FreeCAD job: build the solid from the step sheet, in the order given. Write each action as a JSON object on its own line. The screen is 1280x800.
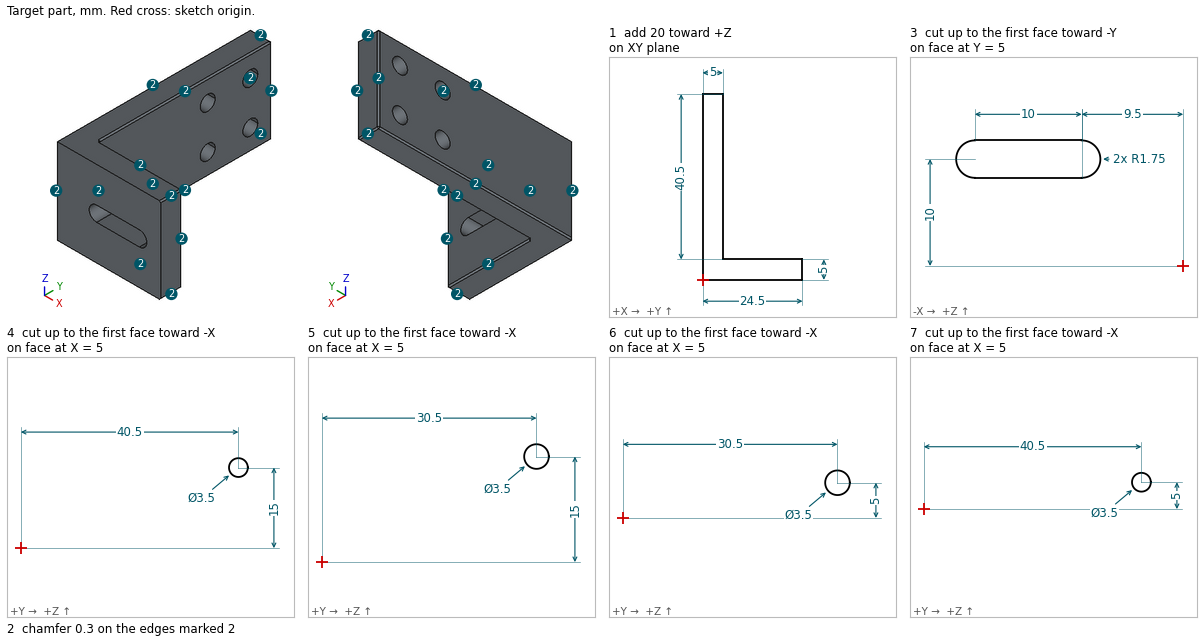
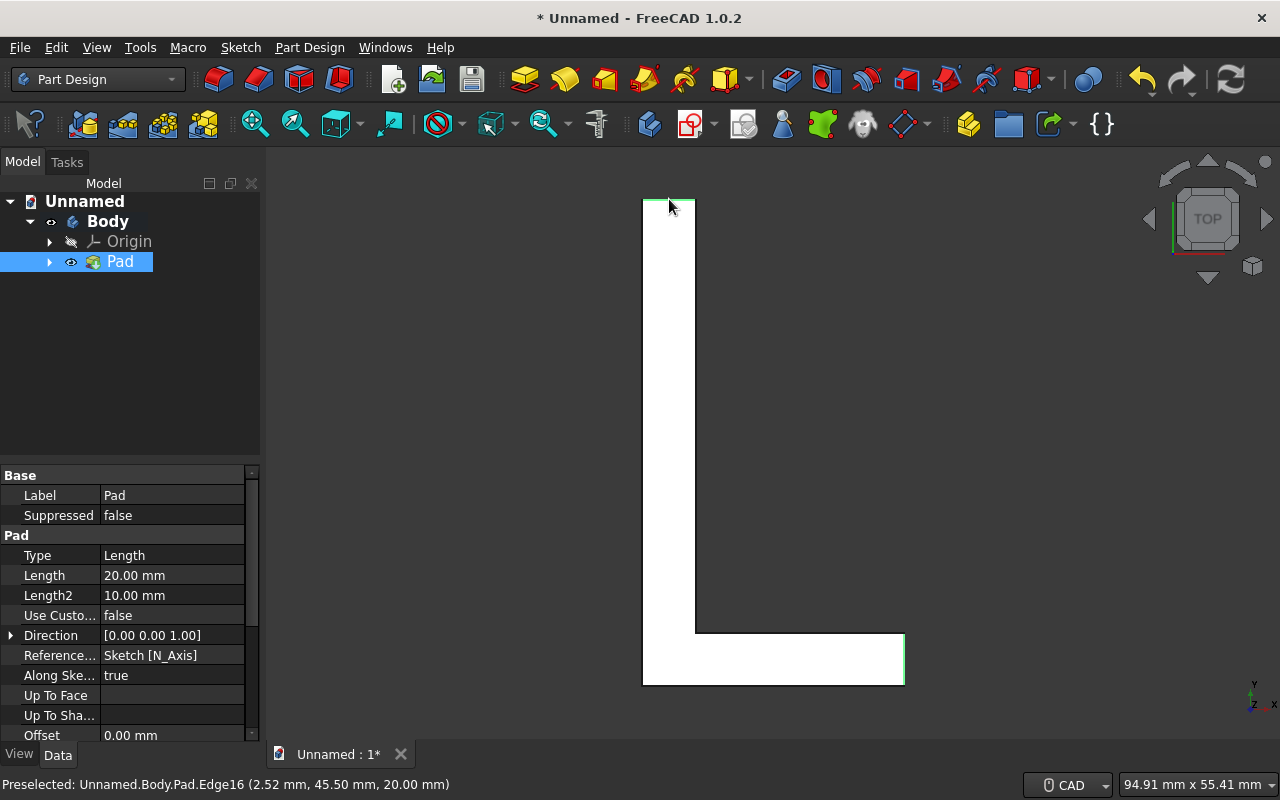
{"action": "key", "text": "1"}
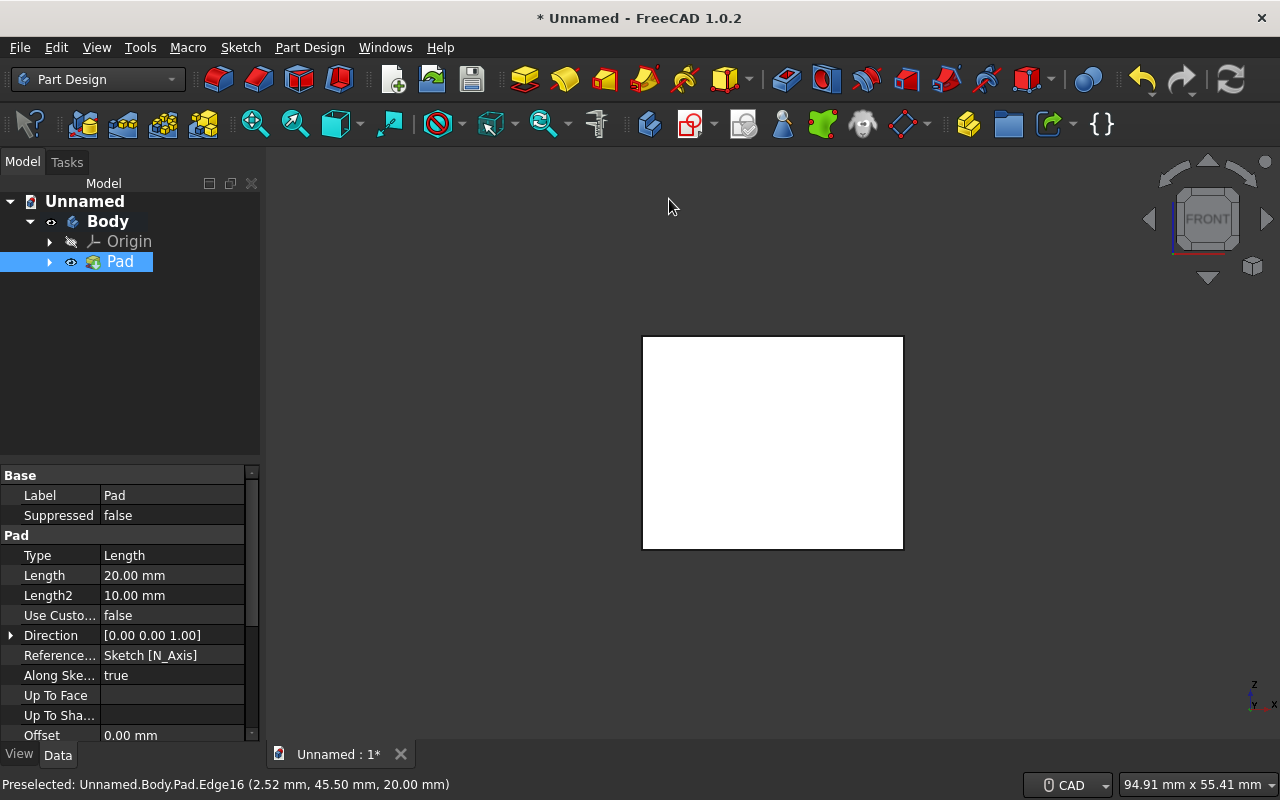
{"action": "left_click", "coordinate": [256, 124]}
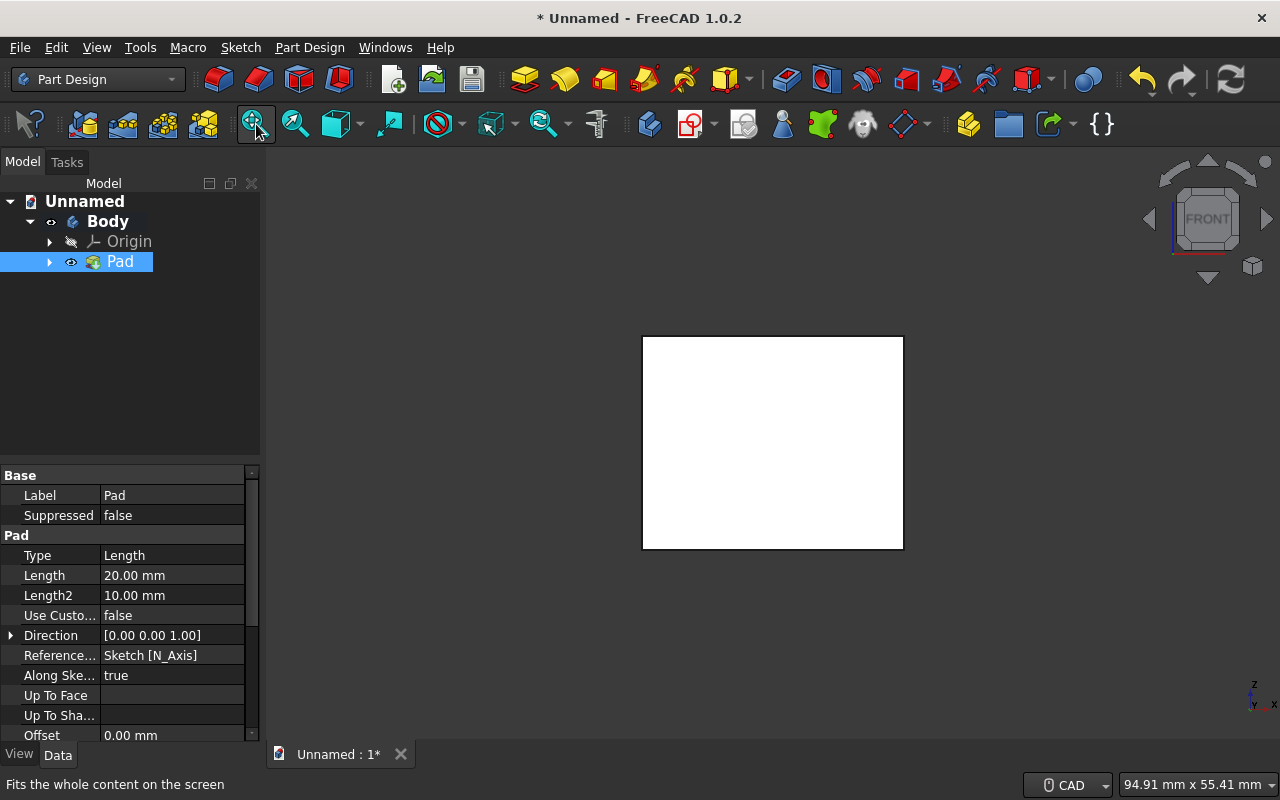
{"action": "key", "text": "3"}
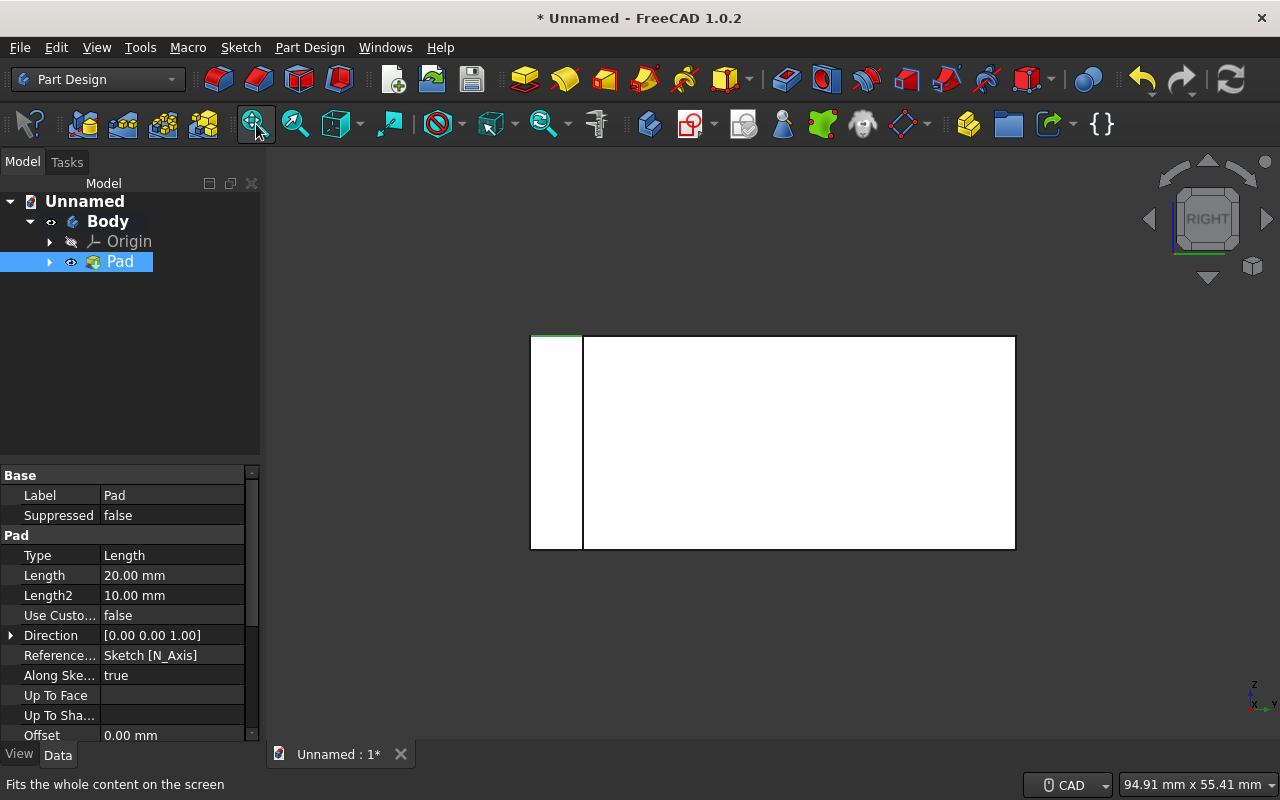
{"action": "left_click", "coordinate": [557, 549], "text": "ctrl"}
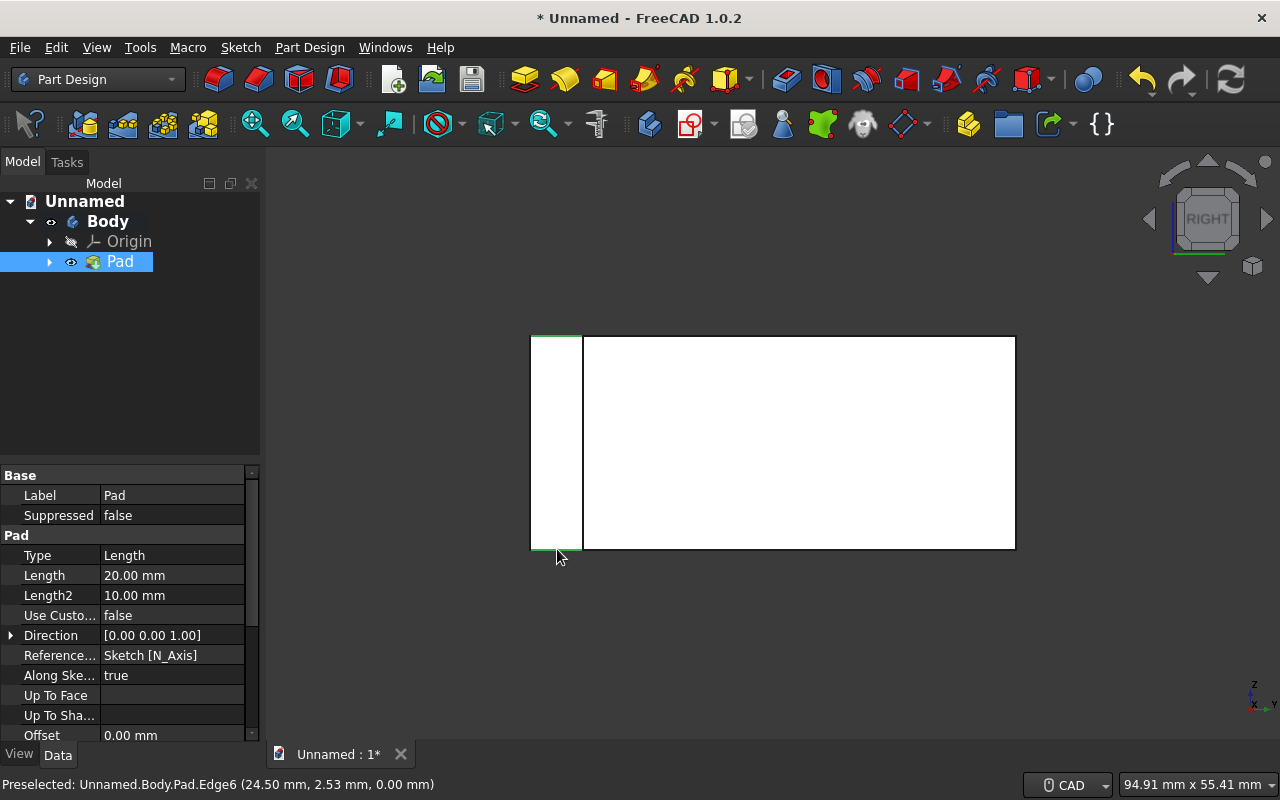
{"action": "key", "text": "5"}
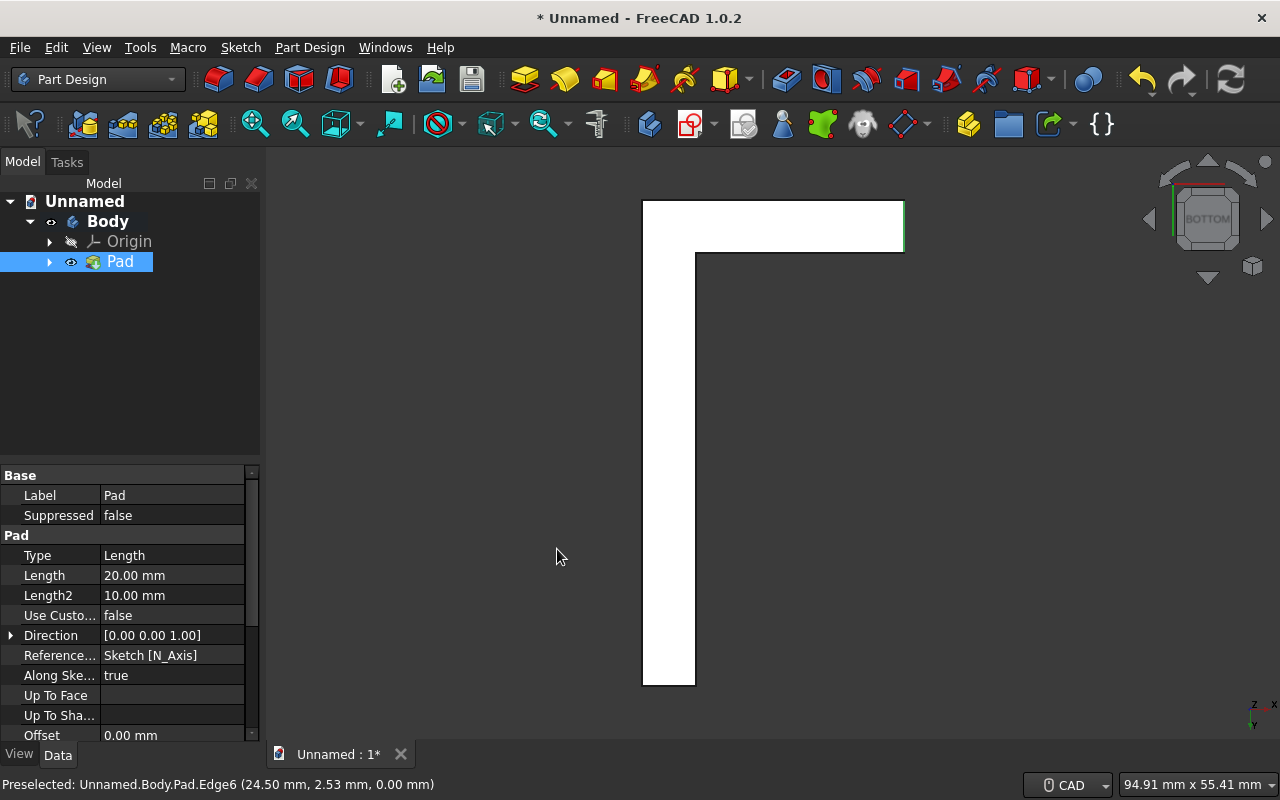
{"action": "left_click", "coordinate": [669, 685], "text": "ctrl"}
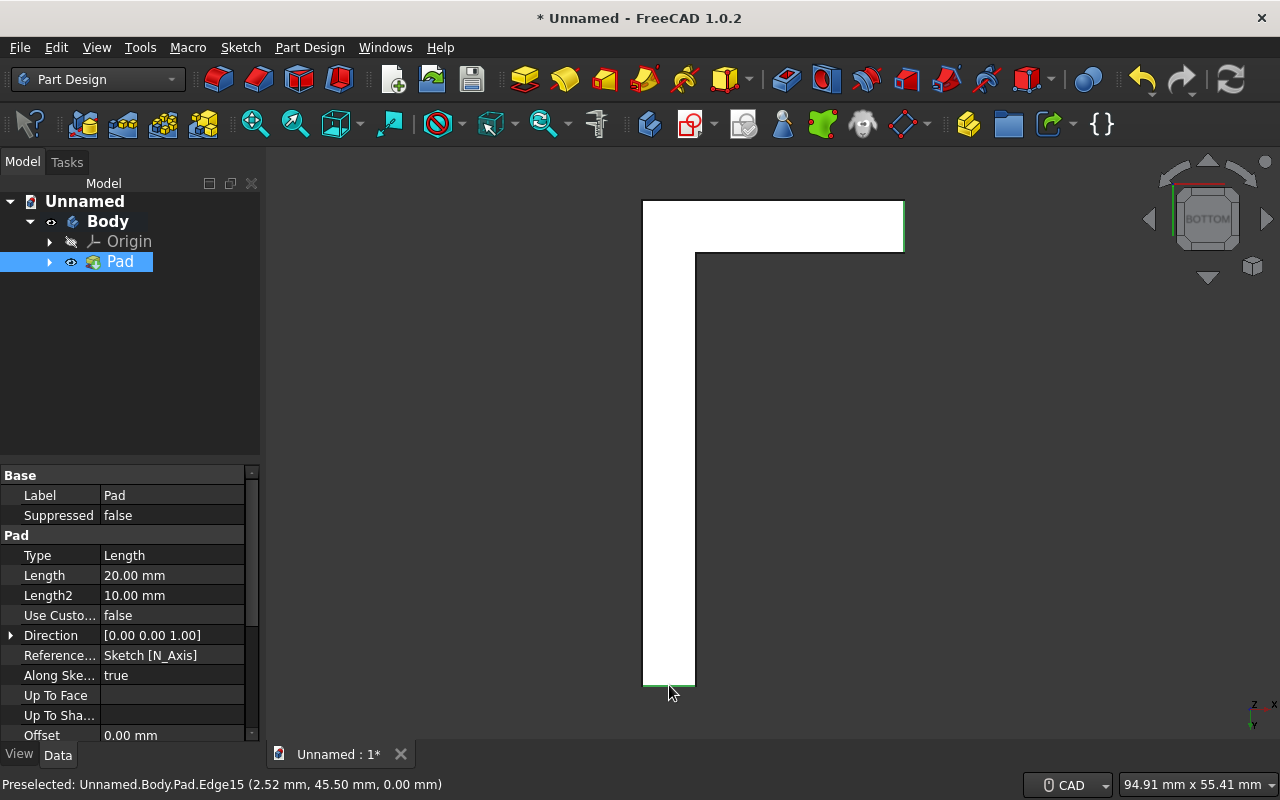
{"action": "key", "text": "4"}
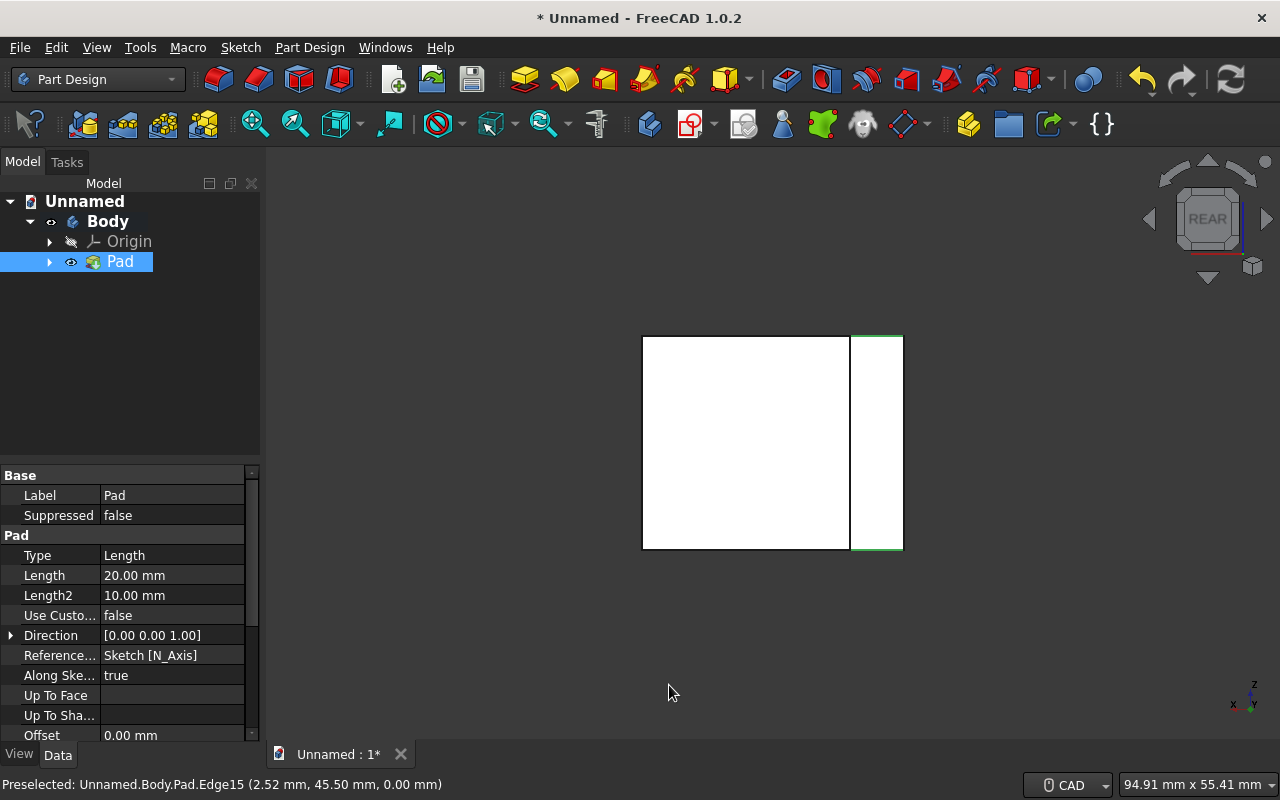
{"action": "key", "text": "v f"}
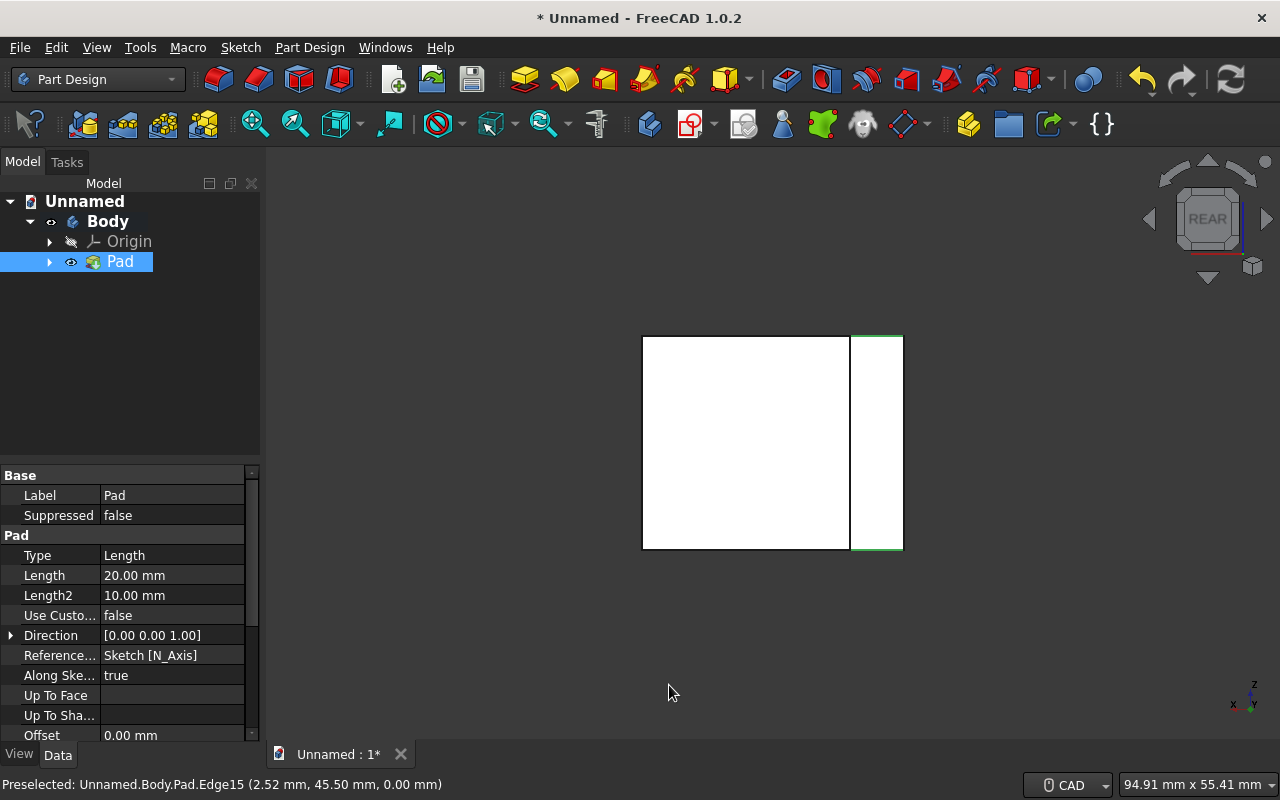
{"action": "left_click", "coordinate": [746, 442], "text": "ctrl"}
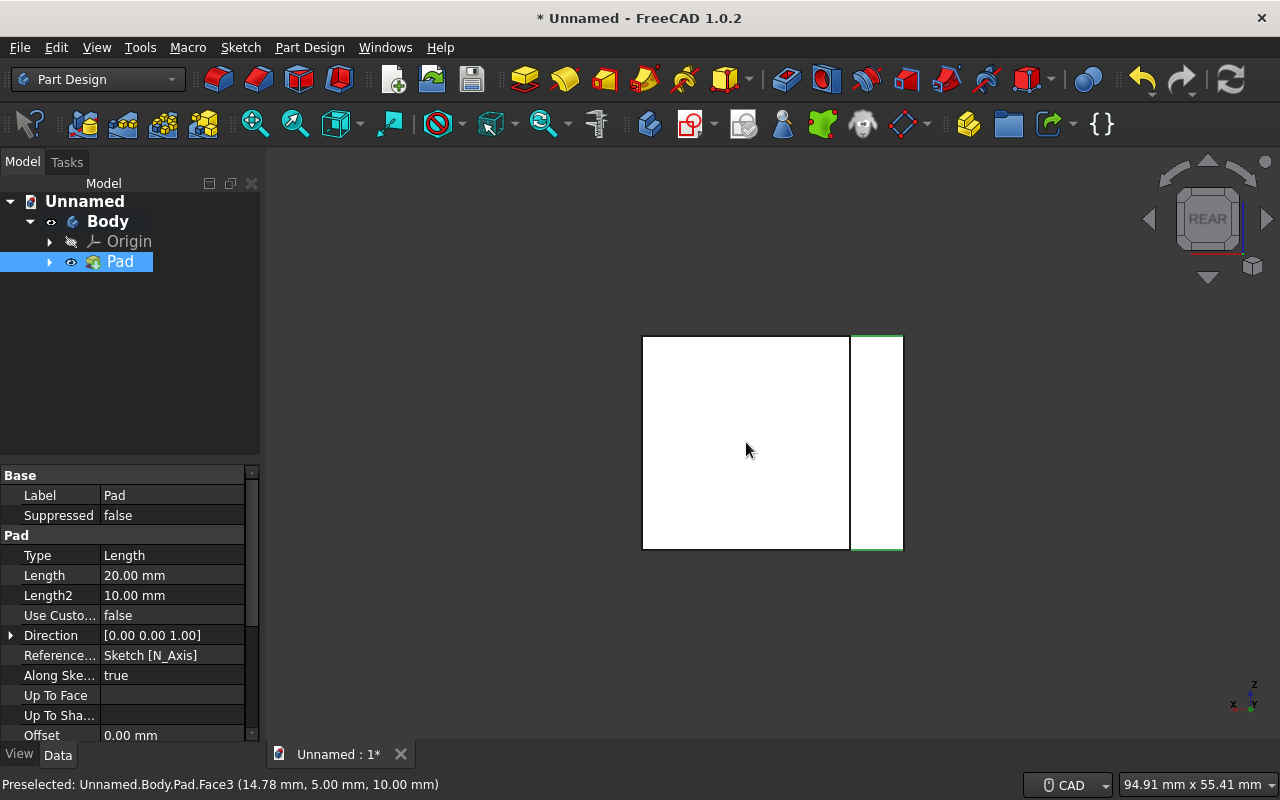
{"action": "key", "text": "6"}